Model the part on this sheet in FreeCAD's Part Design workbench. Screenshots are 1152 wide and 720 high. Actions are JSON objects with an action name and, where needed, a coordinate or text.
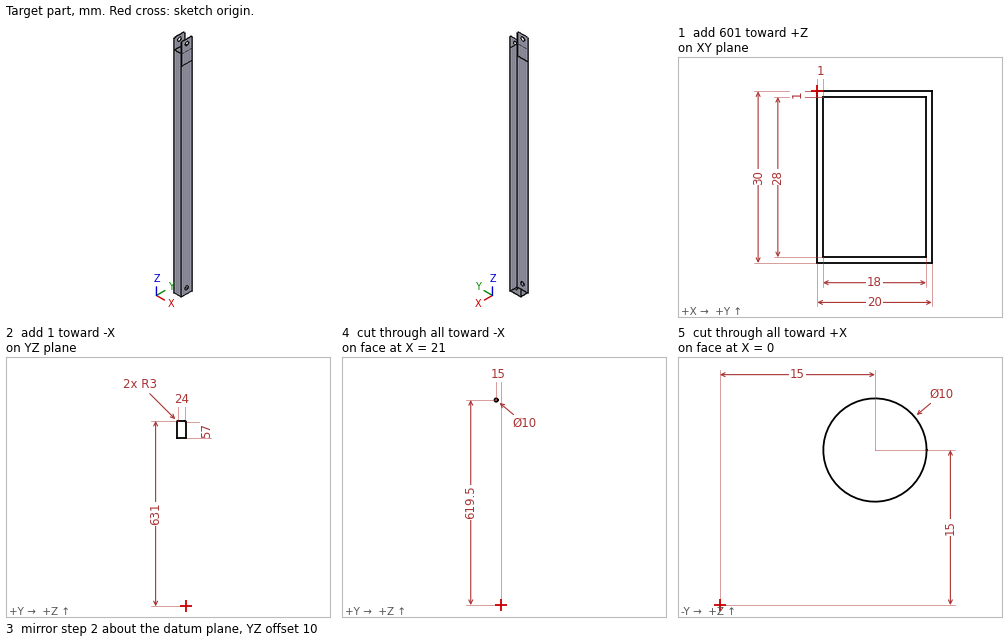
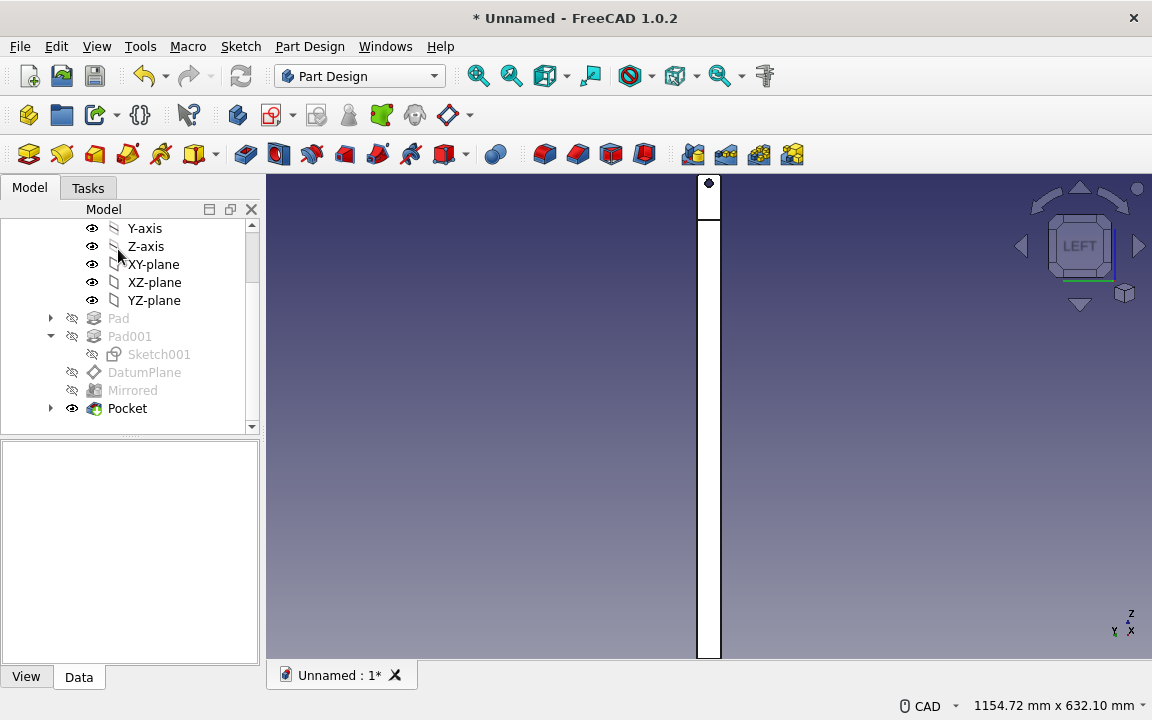
{"action": "left_click", "coordinate": [709, 251]}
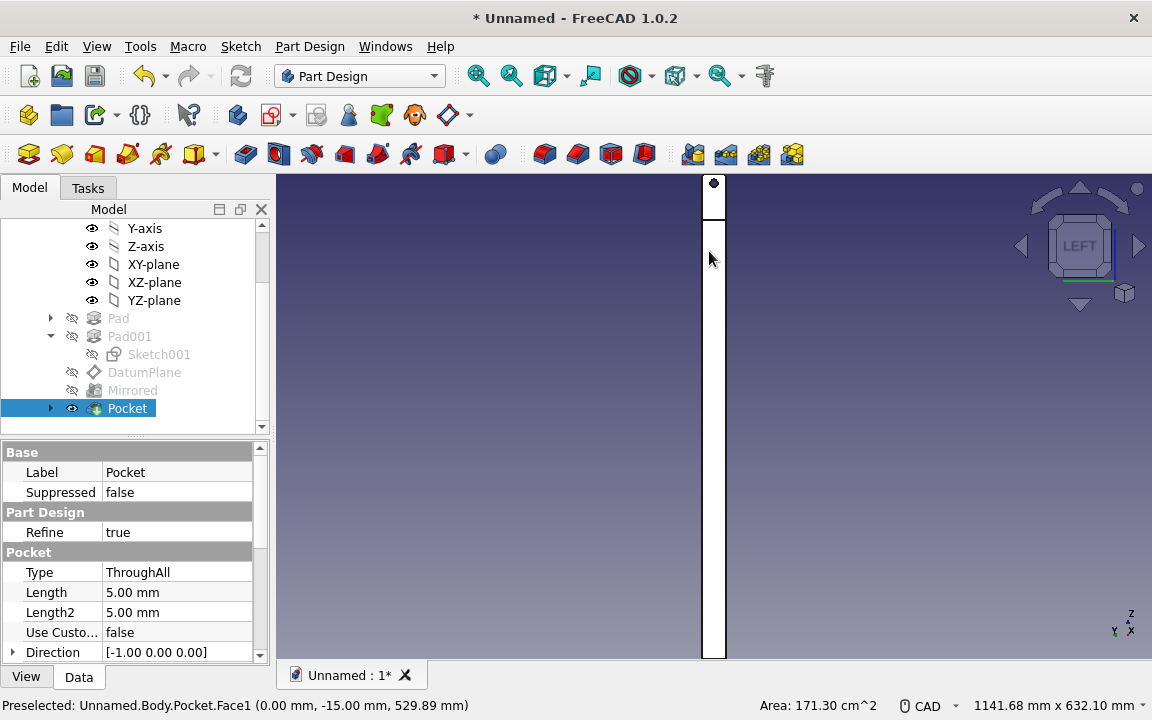
{"action": "left_click", "coordinate": [270, 116]}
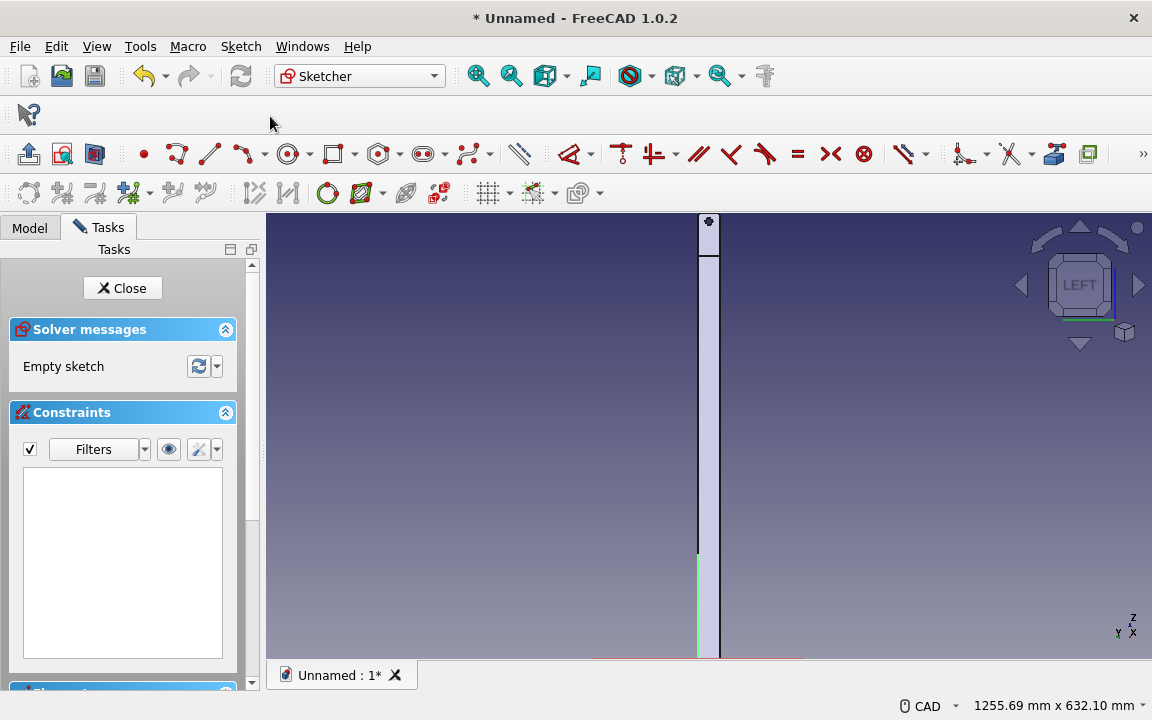
{"action": "scroll", "coordinate": [640, 436], "scroll_direction": "down", "scroll_amount": 5}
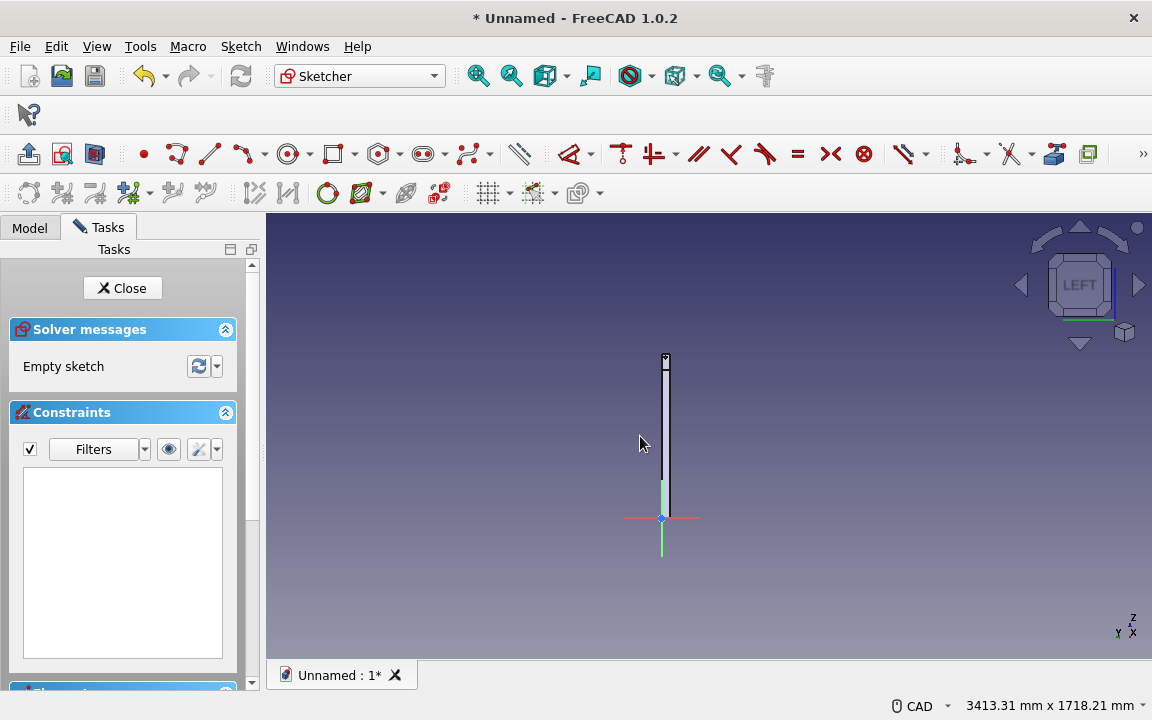
{"action": "scroll", "coordinate": [666, 520], "scroll_direction": "up", "scroll_amount": 15}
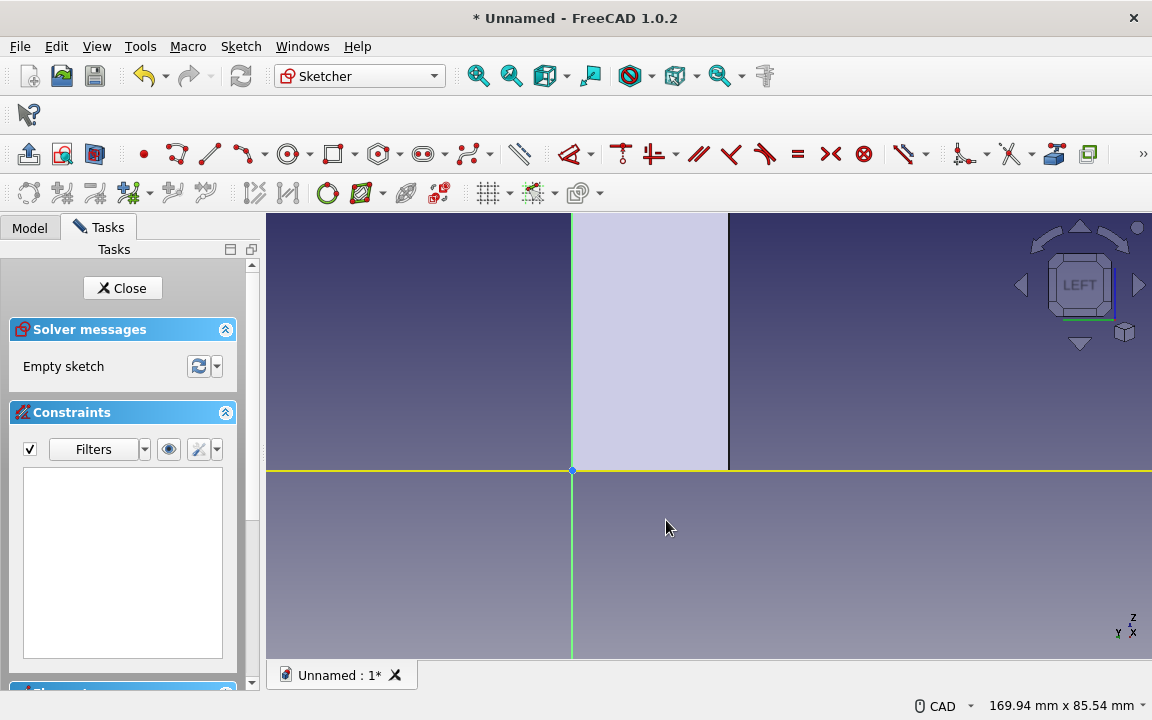
{"action": "scroll", "coordinate": [615, 409], "scroll_direction": "up", "scroll_amount": 5}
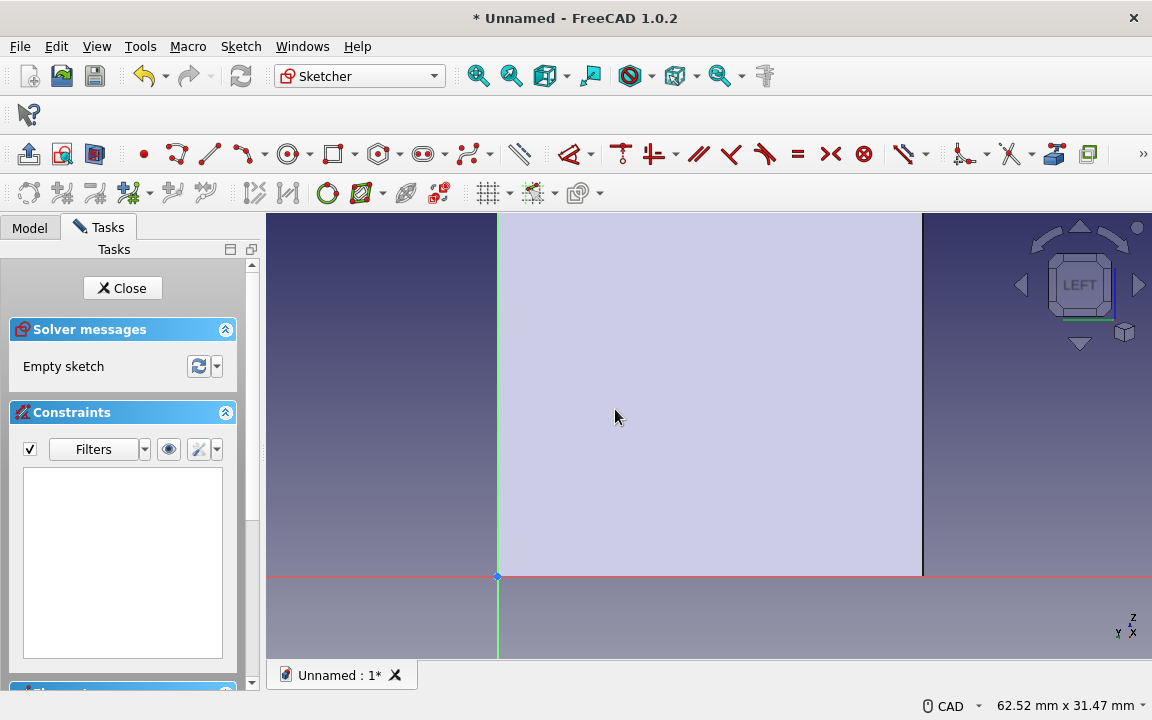
{"action": "key", "text": "g c"}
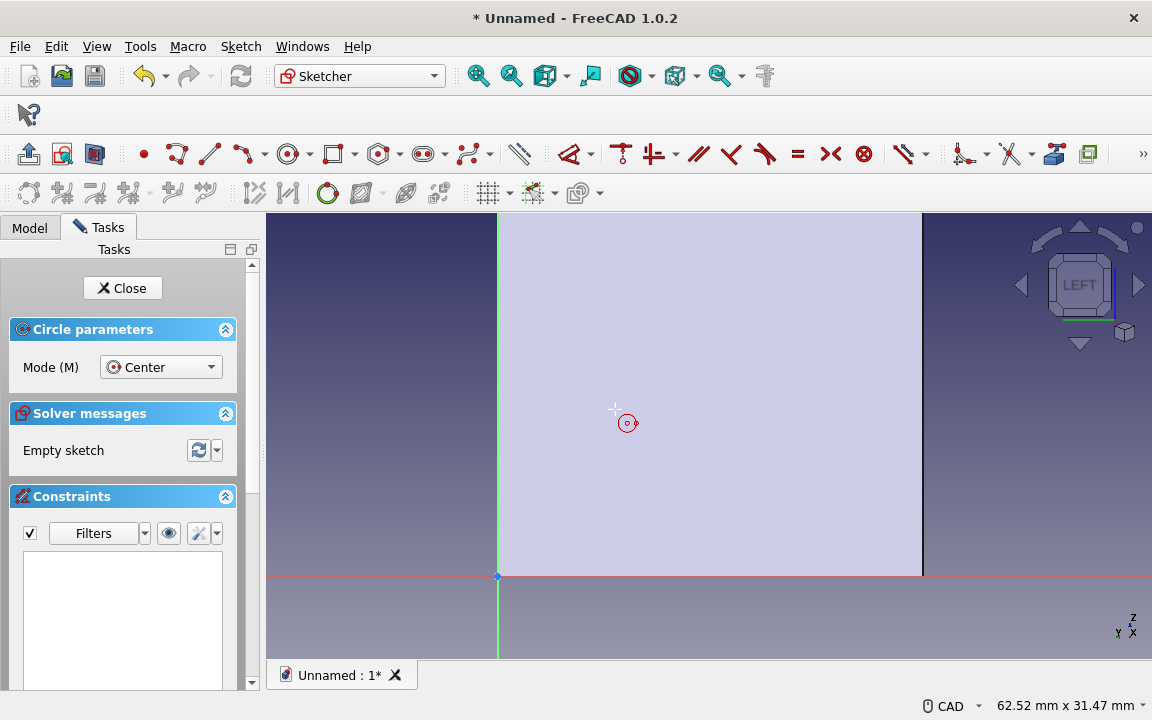
{"action": "left_click", "coordinate": [710, 364]}
{"action": "left_click", "coordinate": [761, 314]}
{"action": "key", "text": "Escape"}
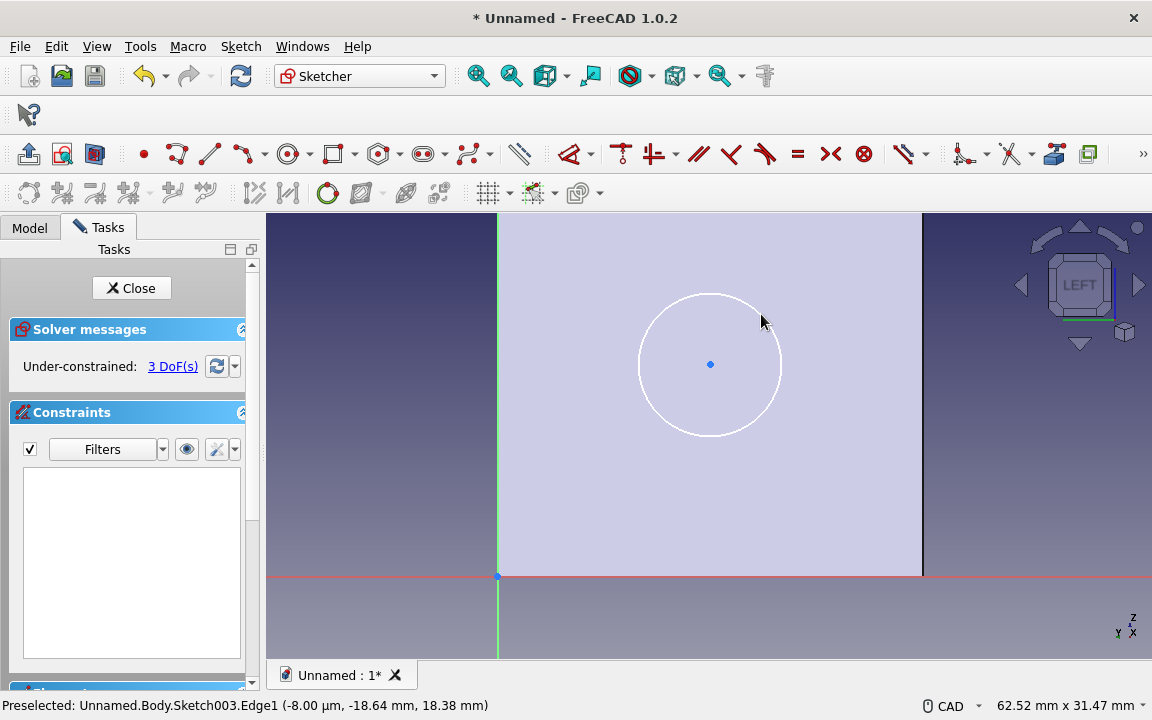
{"action": "key", "text": "d"}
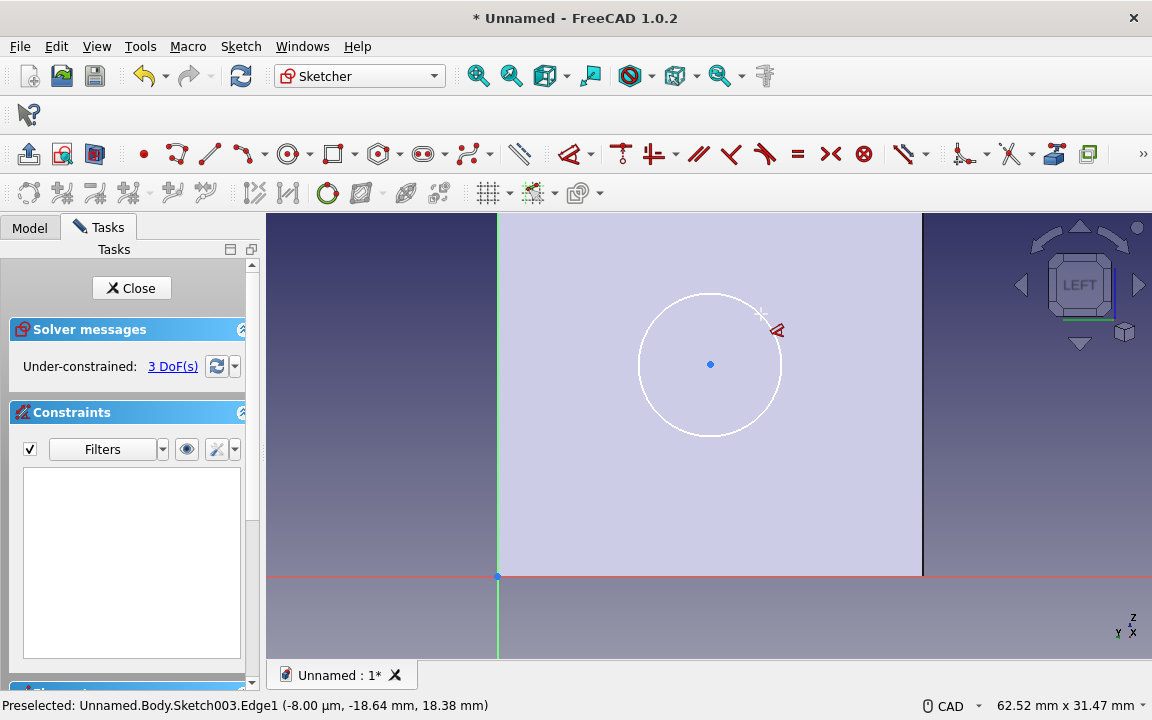
{"action": "left_click", "coordinate": [760, 314]}
{"action": "left_click", "coordinate": [782, 291]}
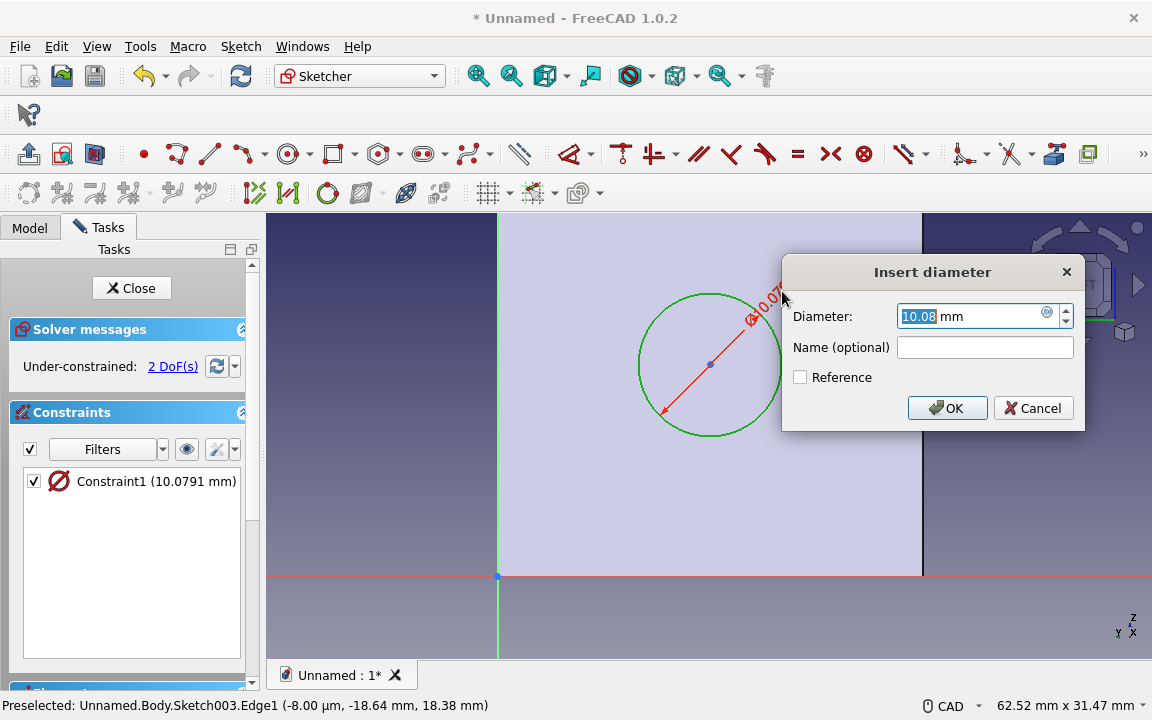
{"action": "type", "text": "10"}
{"action": "key", "text": "Return"}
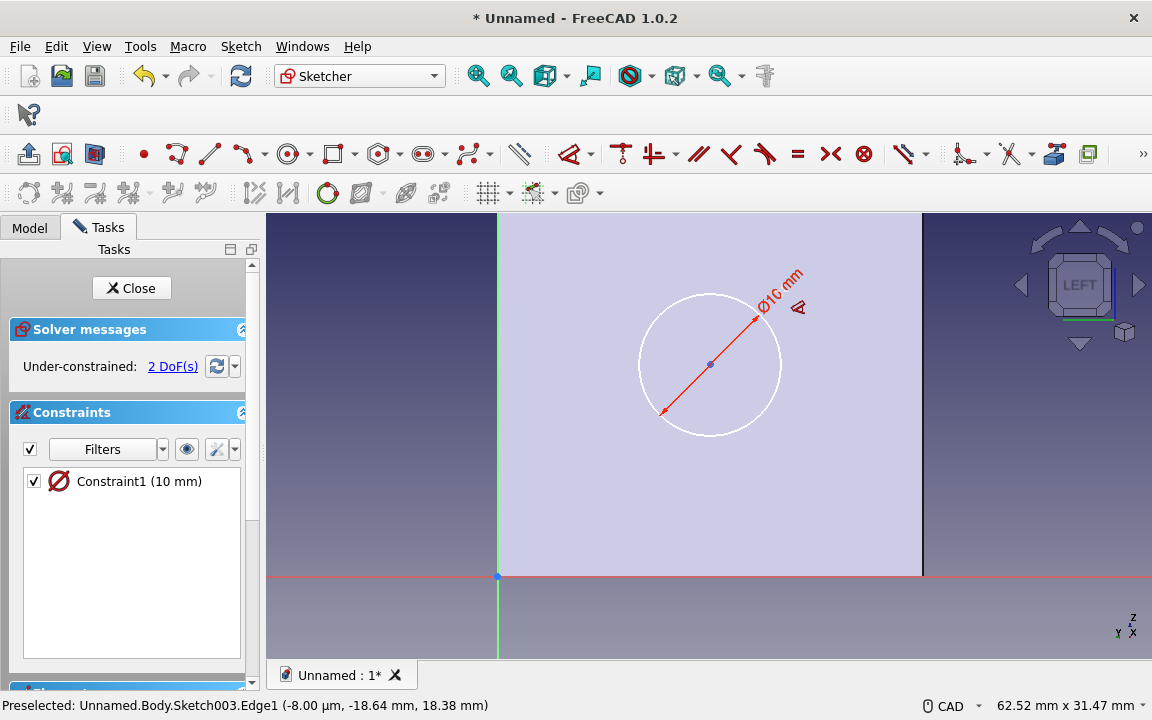
{"action": "left_click", "coordinate": [710, 365]}
{"action": "left_click", "coordinate": [604, 611]}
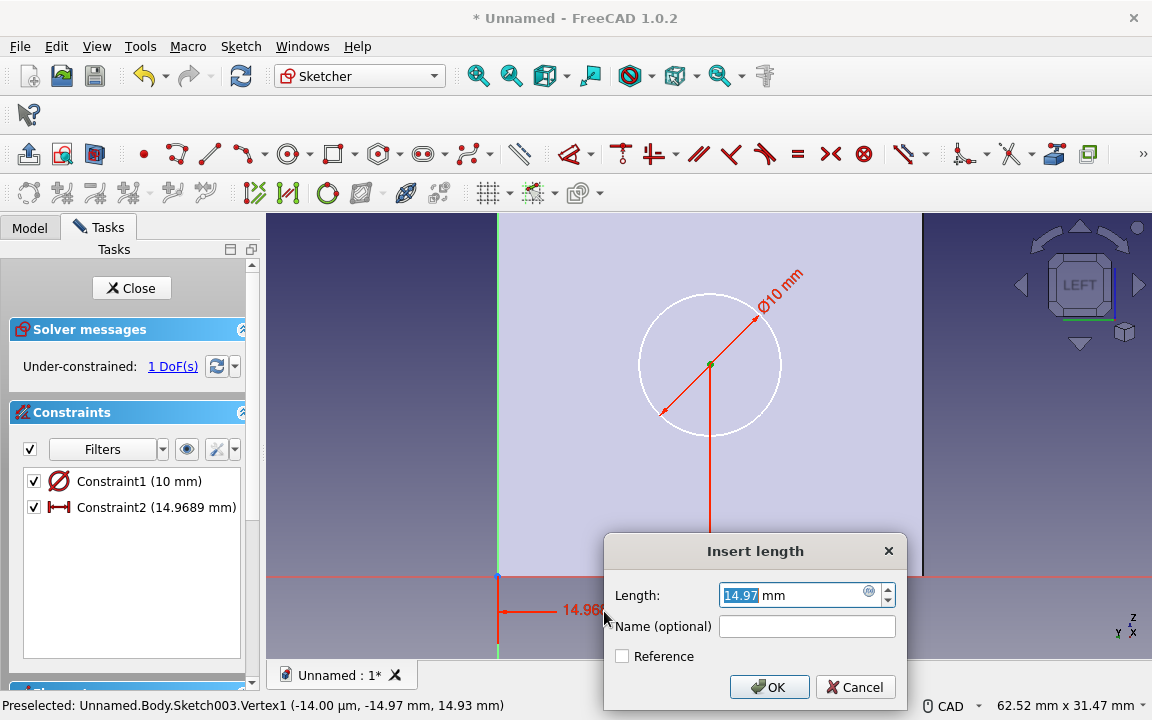
{"action": "type", "text": "15"}
{"action": "key", "text": "Return"}